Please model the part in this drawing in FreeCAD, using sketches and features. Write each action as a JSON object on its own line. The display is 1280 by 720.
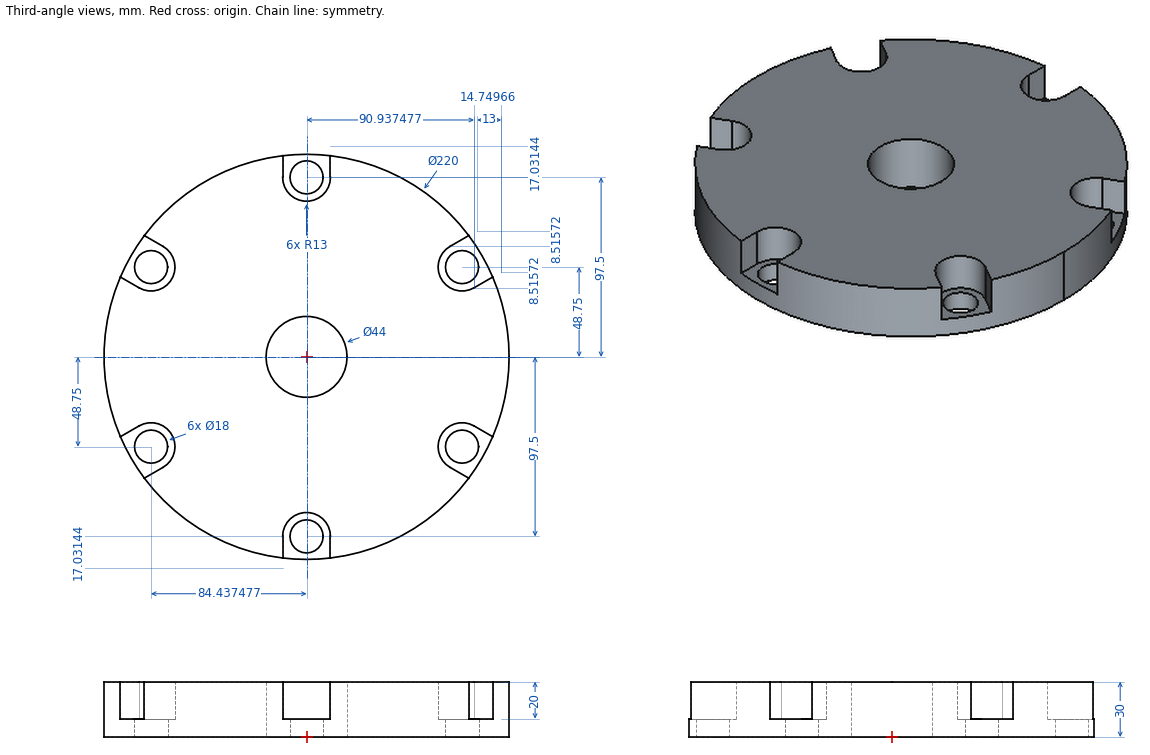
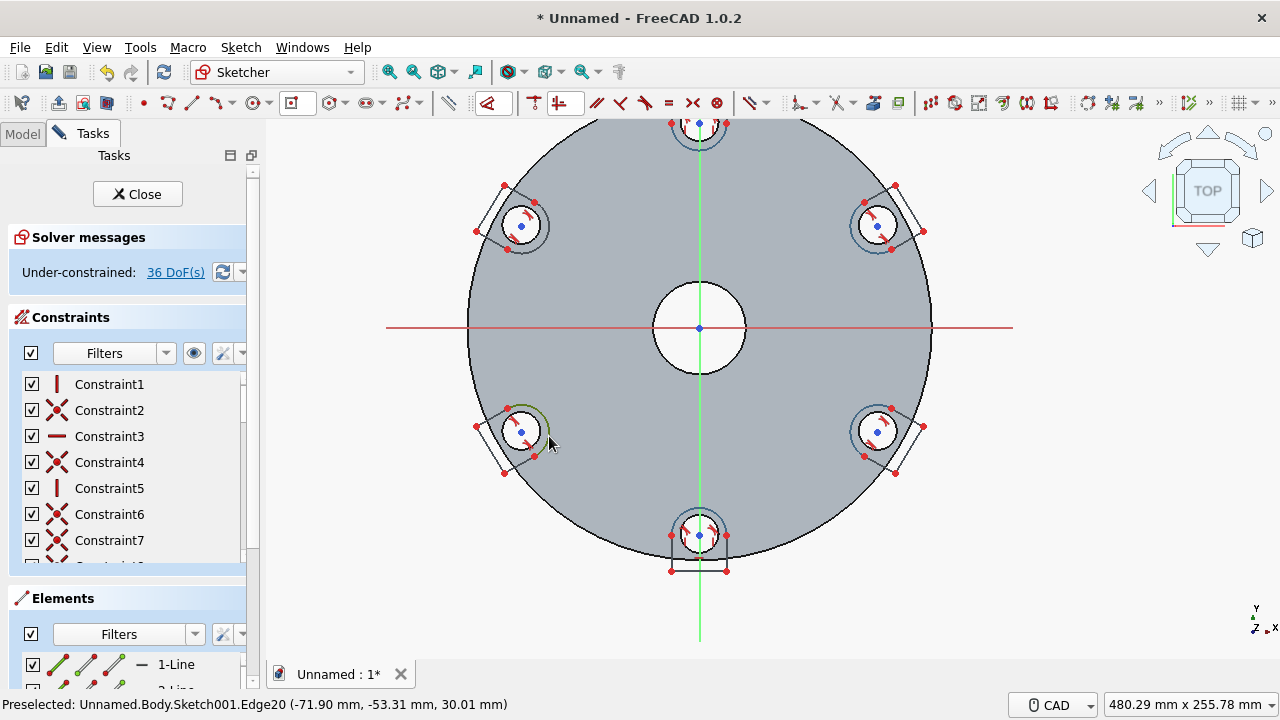
{"action": "left_click", "coordinate": [533, 251]}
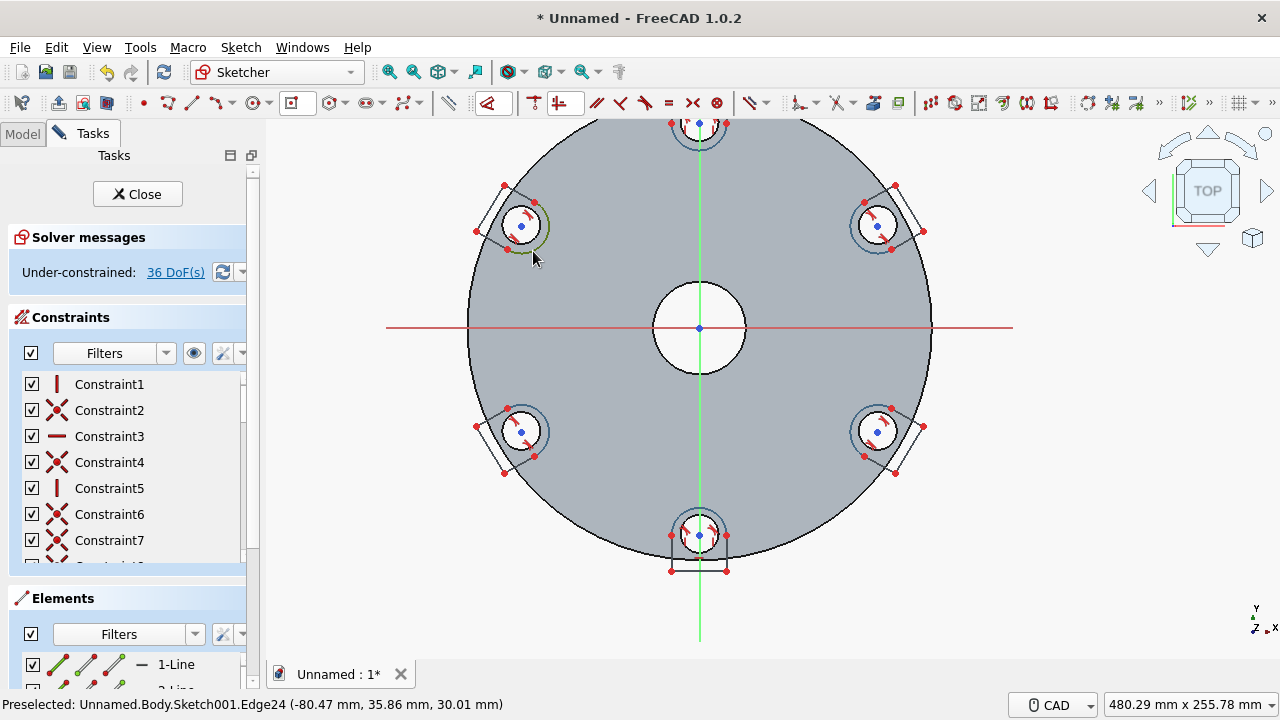
{"action": "left_click", "coordinate": [670, 104]}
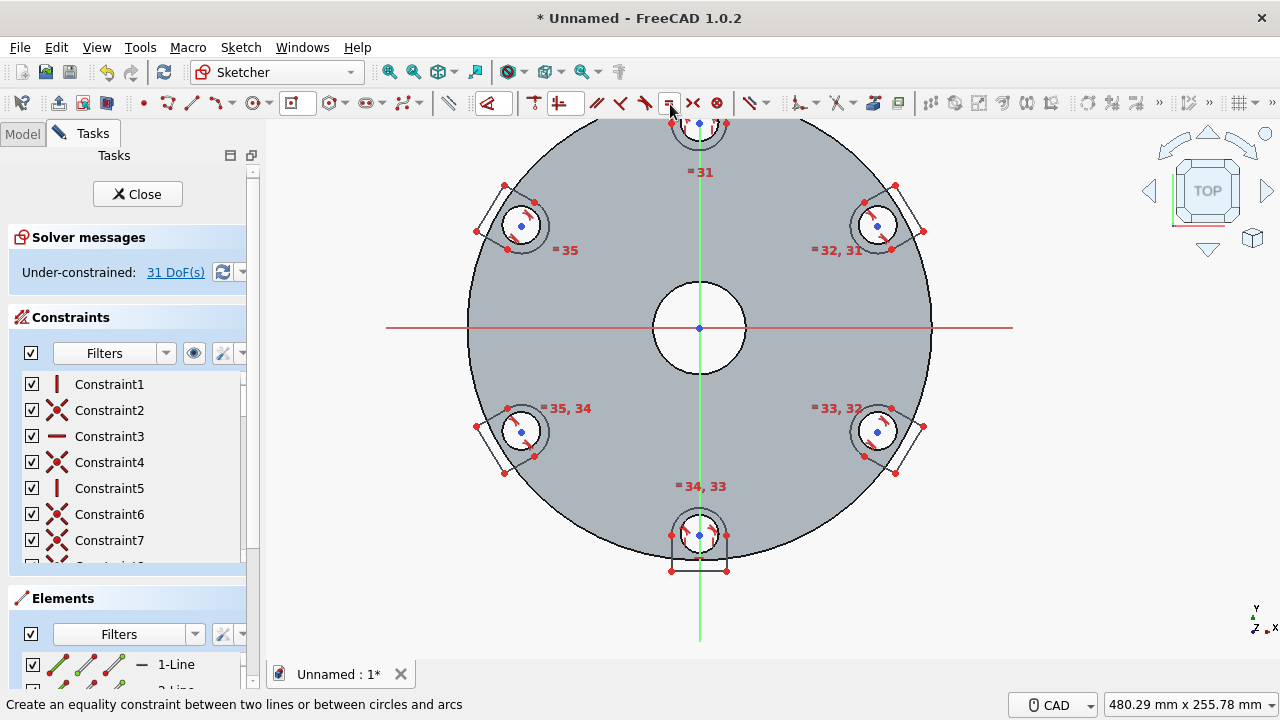
{"action": "scroll", "coordinate": [715, 513], "scroll_direction": "down", "scroll_amount": 2}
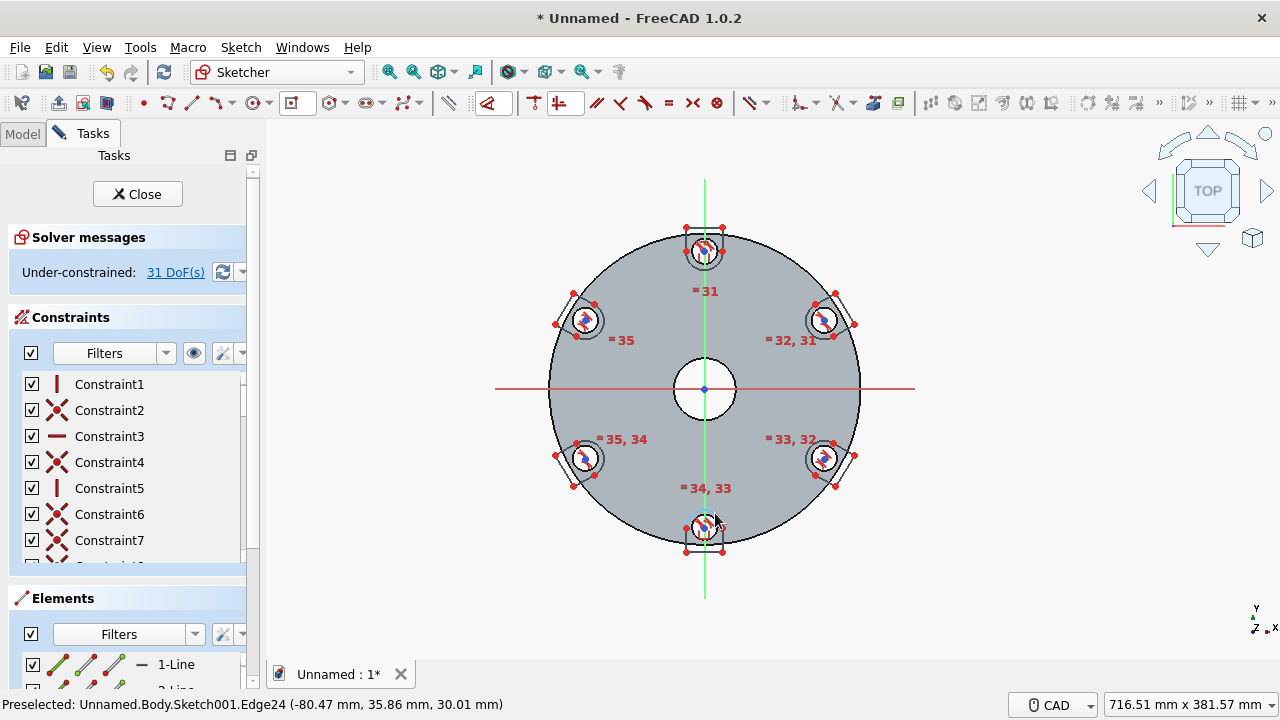
{"action": "left_click", "coordinate": [704, 252]}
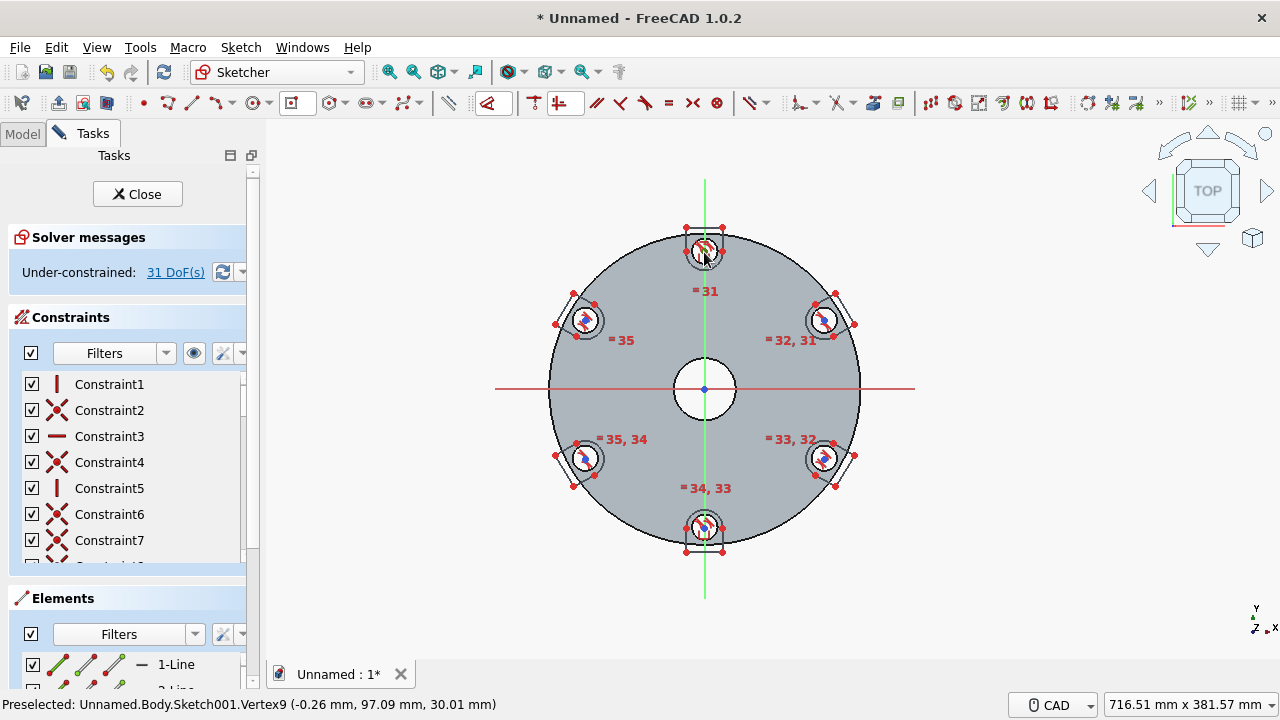
{"action": "left_click", "coordinate": [705, 596]}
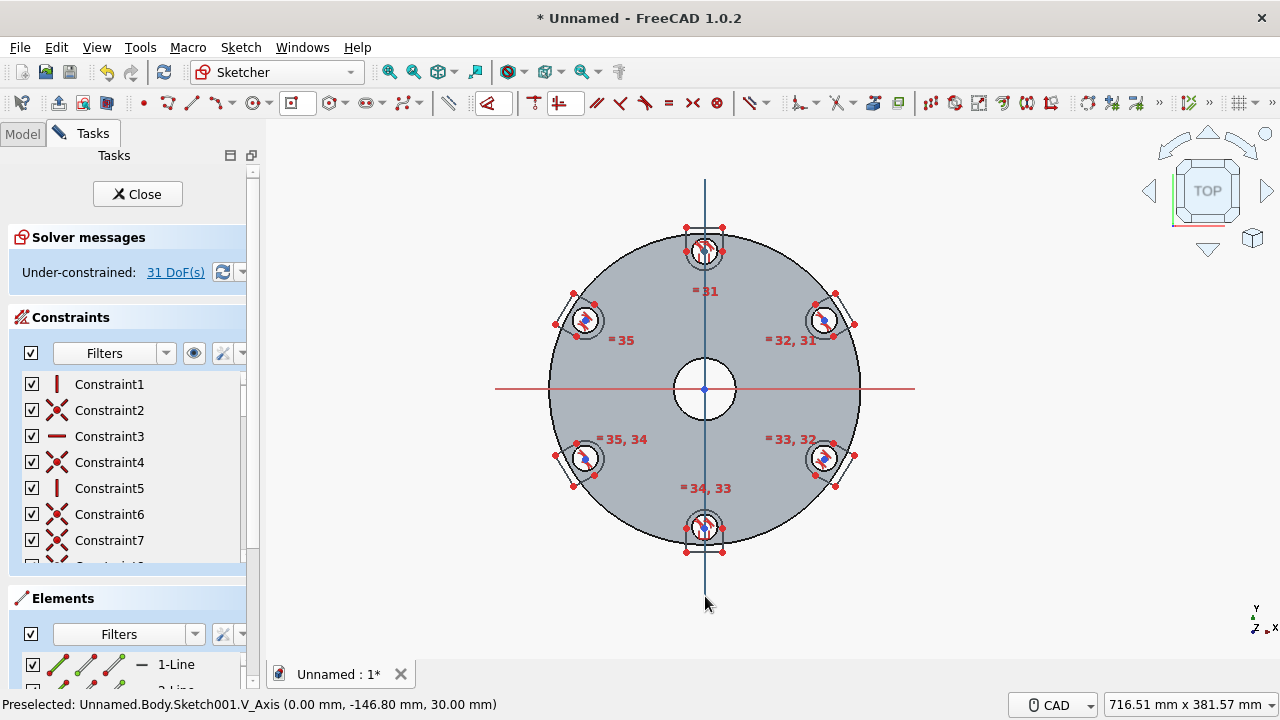
{"action": "left_click", "coordinate": [534, 104]}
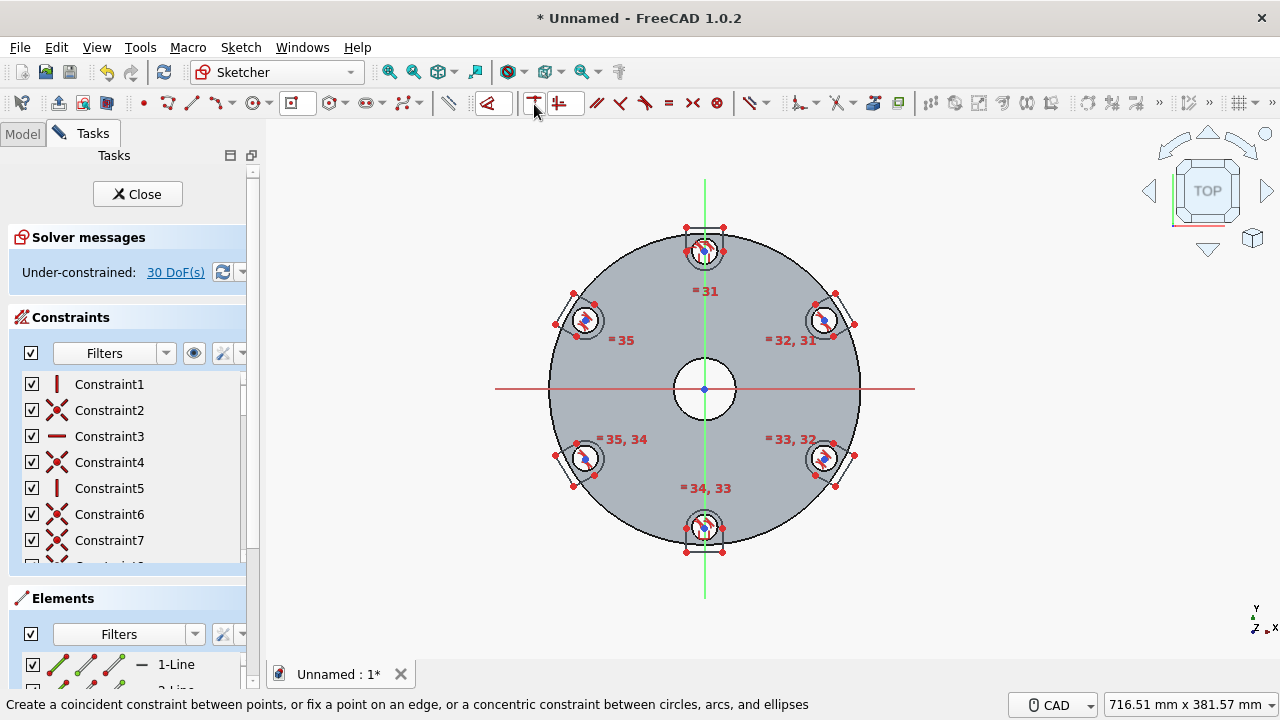
{"action": "left_click", "coordinate": [705, 528]}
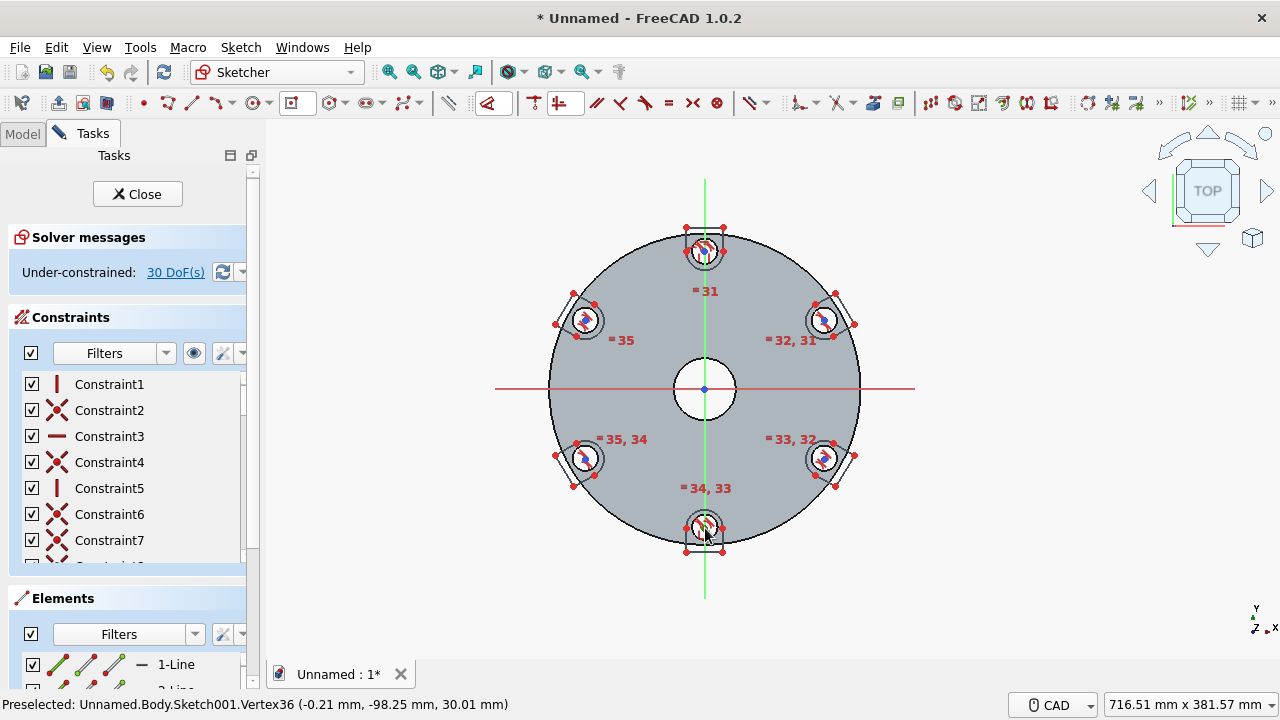
{"action": "left_click", "coordinate": [705, 596]}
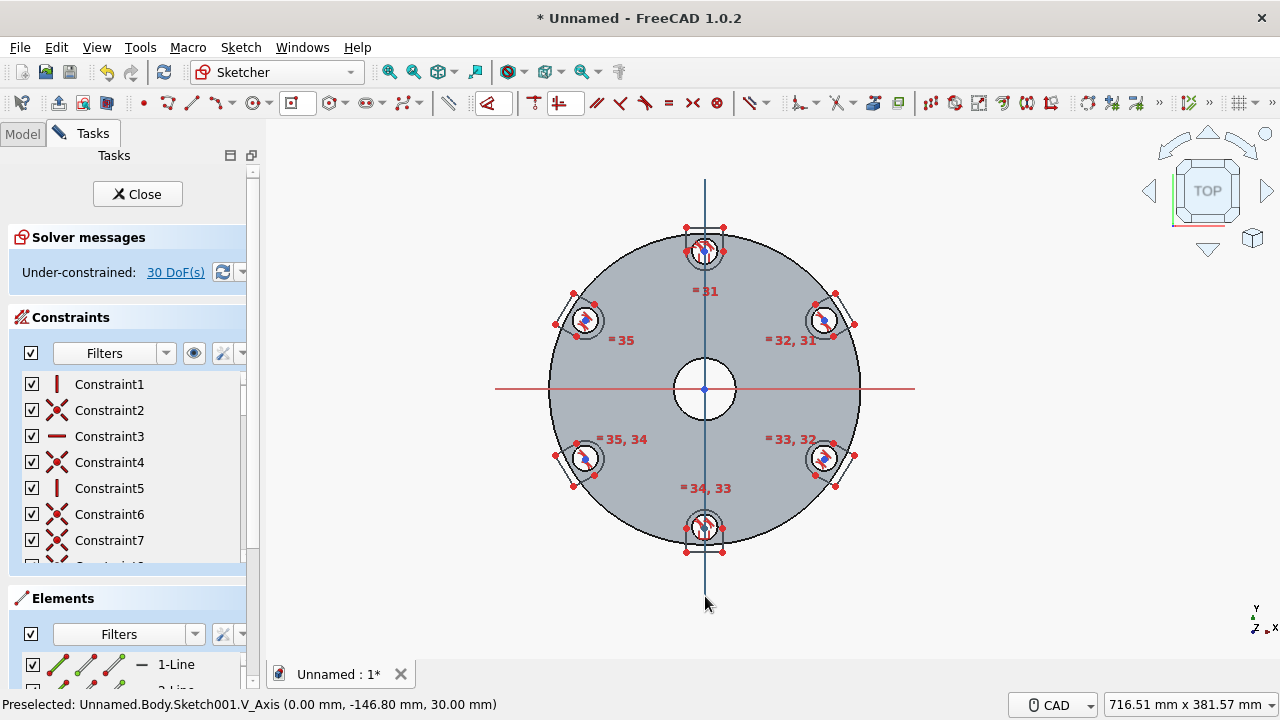
{"action": "left_click", "coordinate": [534, 104]}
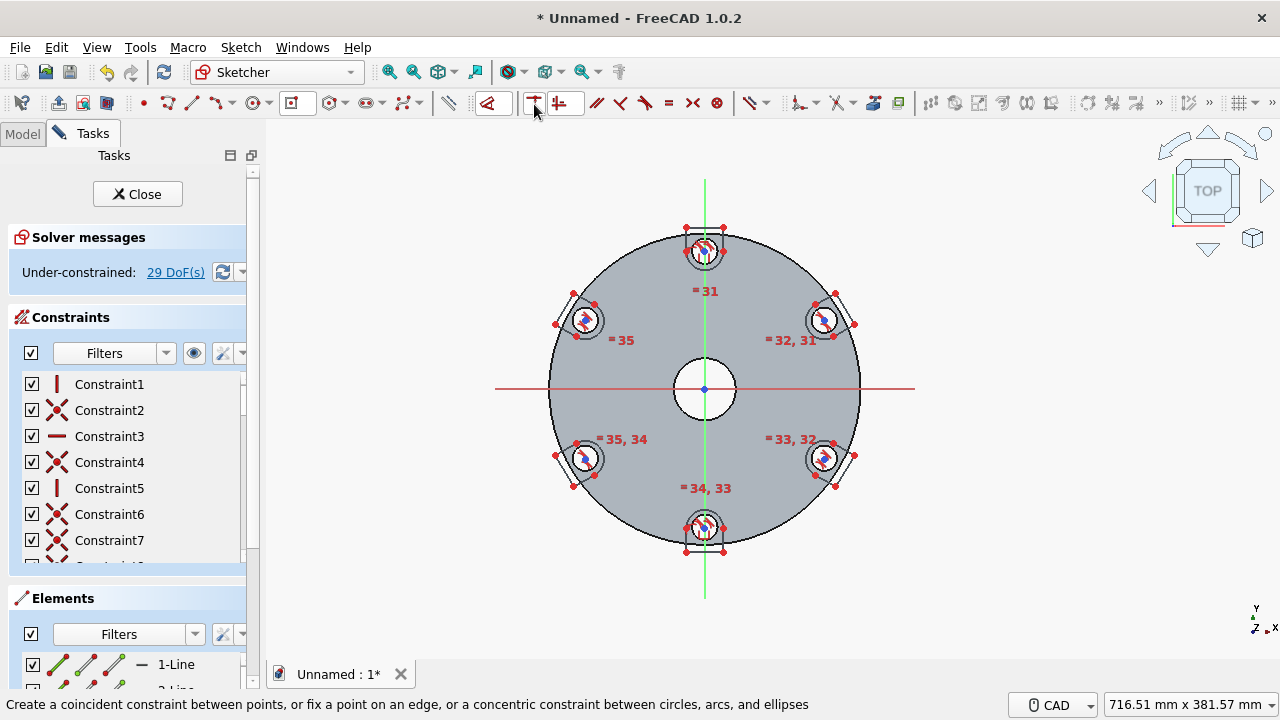
{"action": "left_click", "coordinate": [824, 321]}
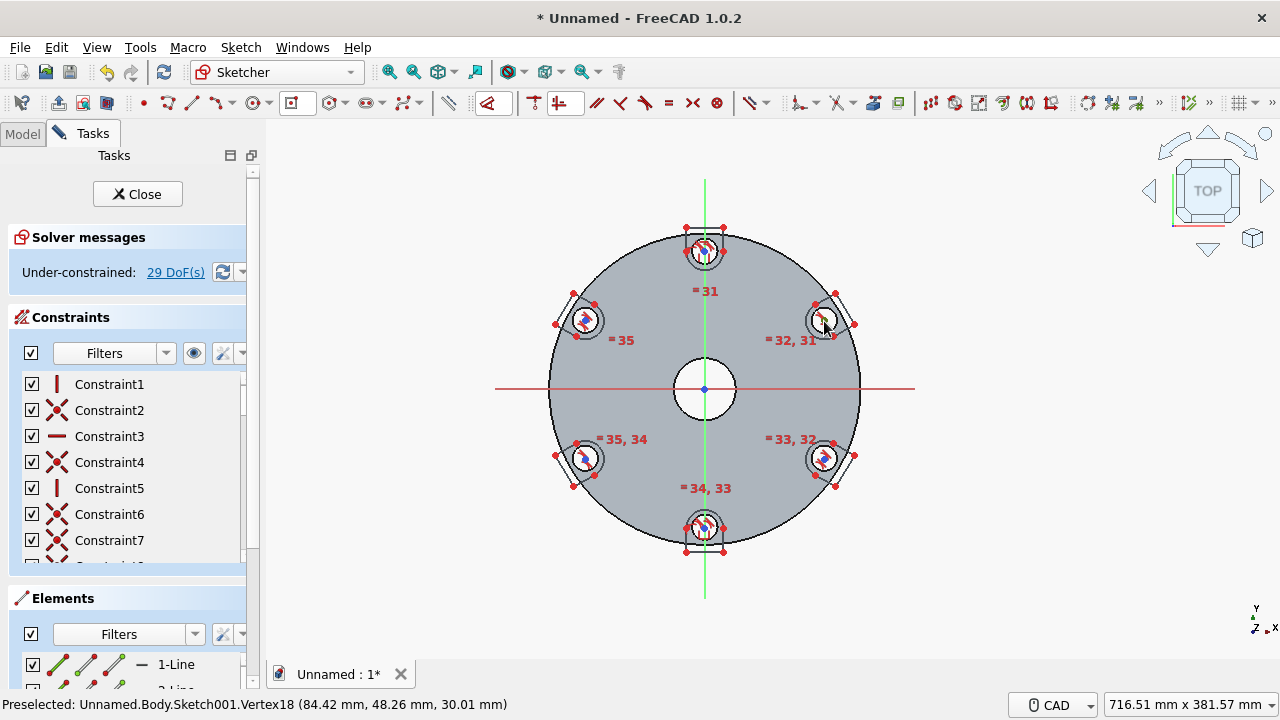
{"action": "left_click", "coordinate": [824, 459]}